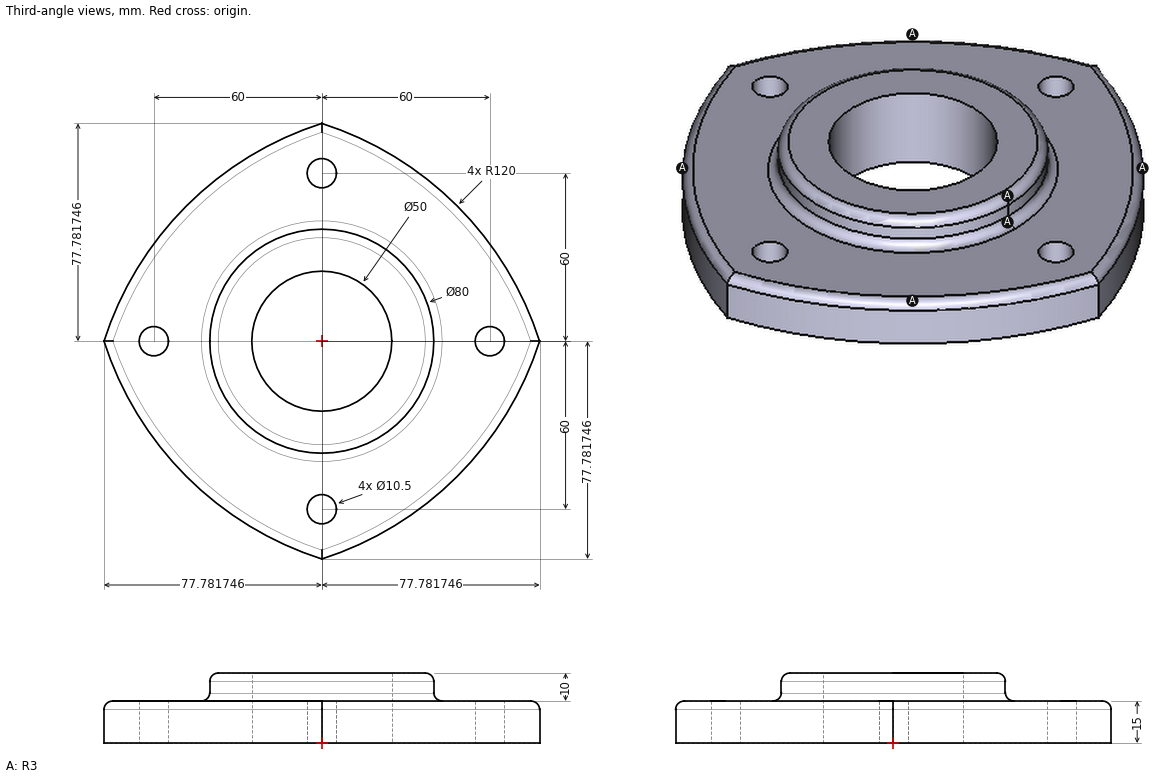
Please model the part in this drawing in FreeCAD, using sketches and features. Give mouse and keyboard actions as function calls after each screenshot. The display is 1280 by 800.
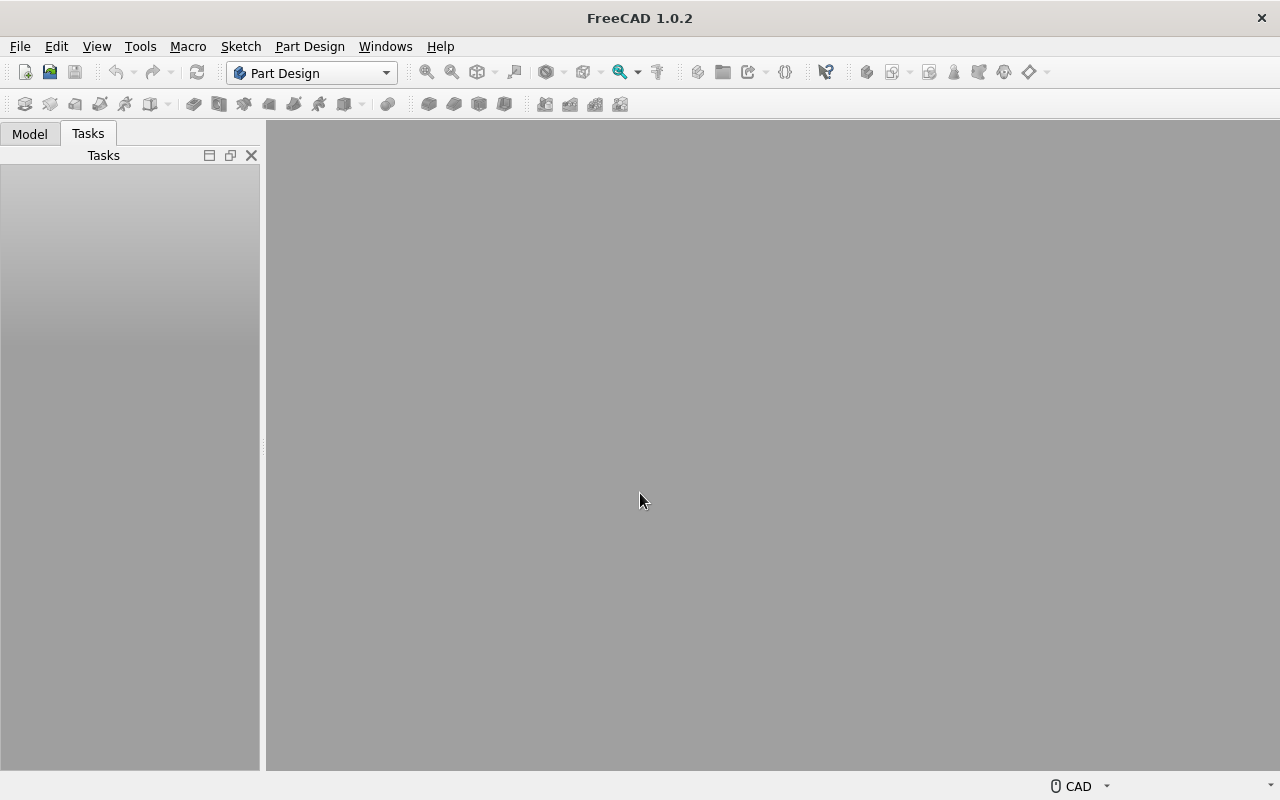
click(25, 72)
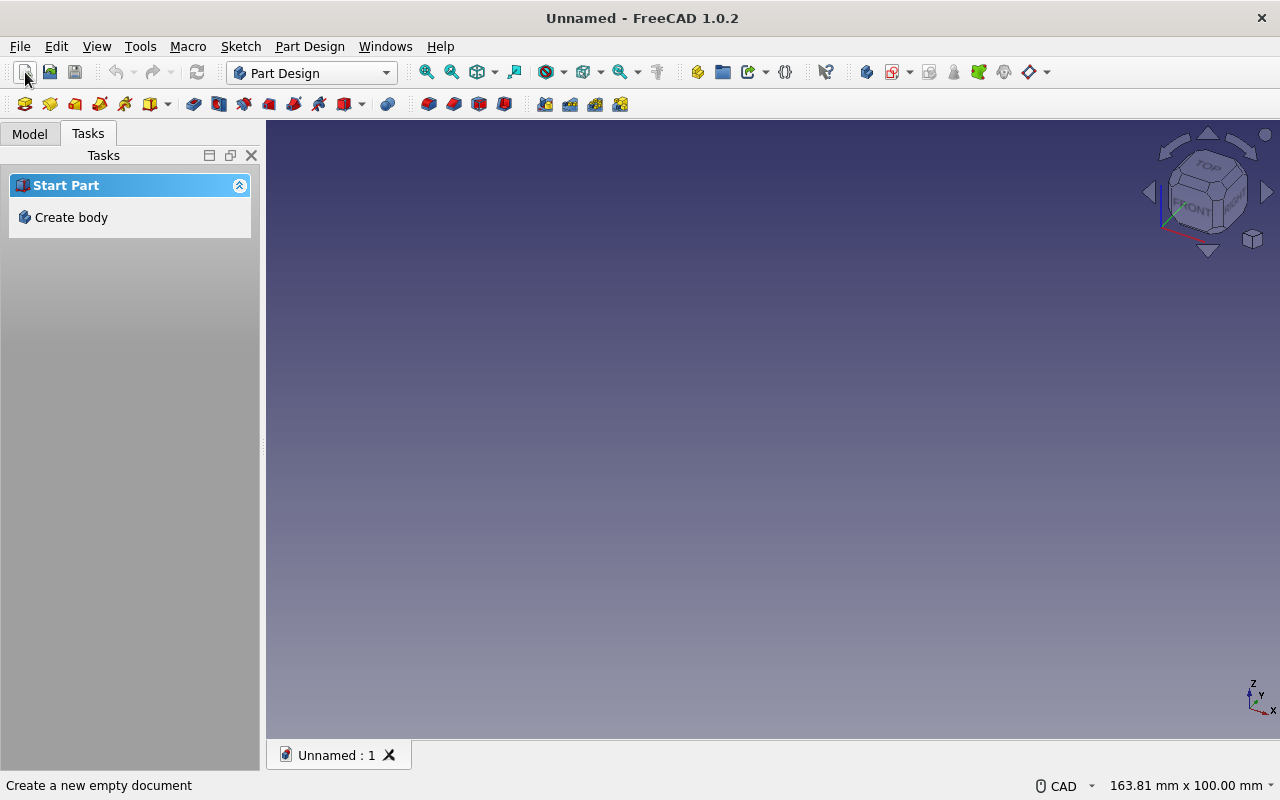
click(892, 72)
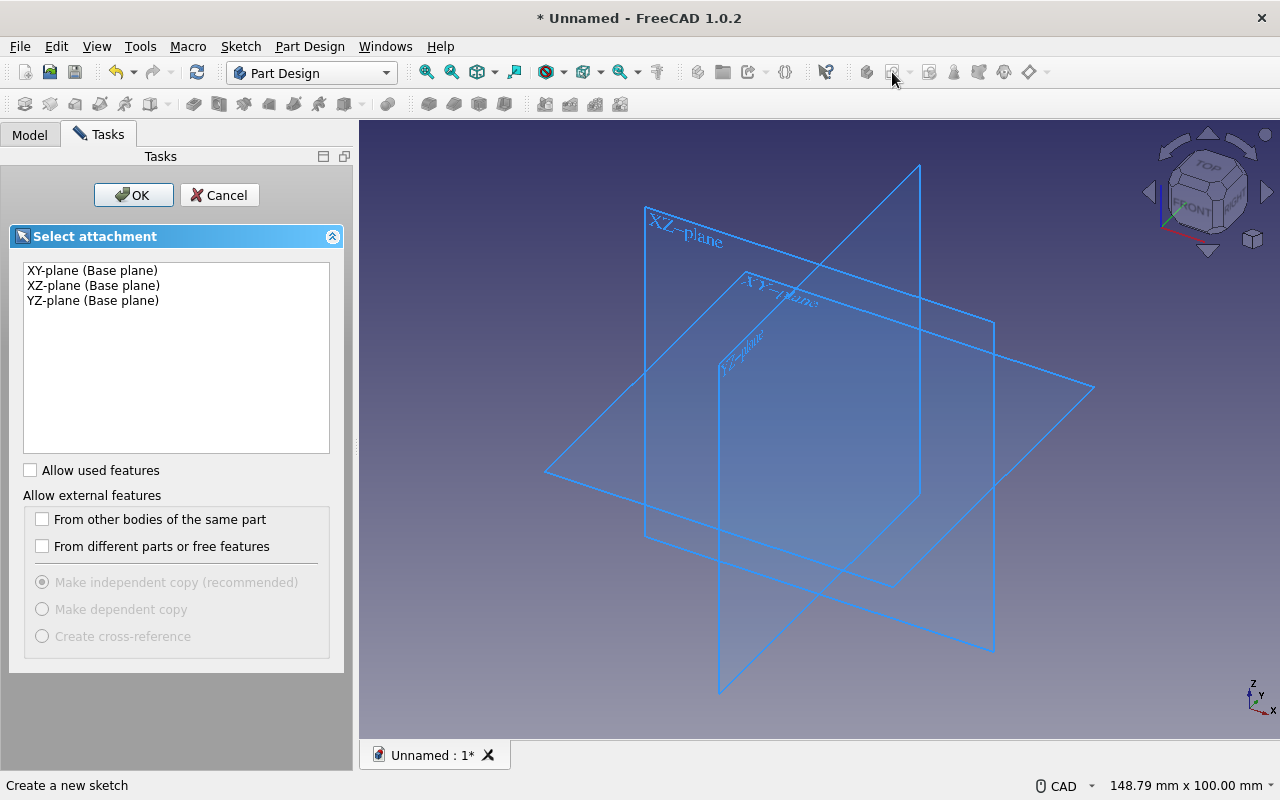
click(84, 270)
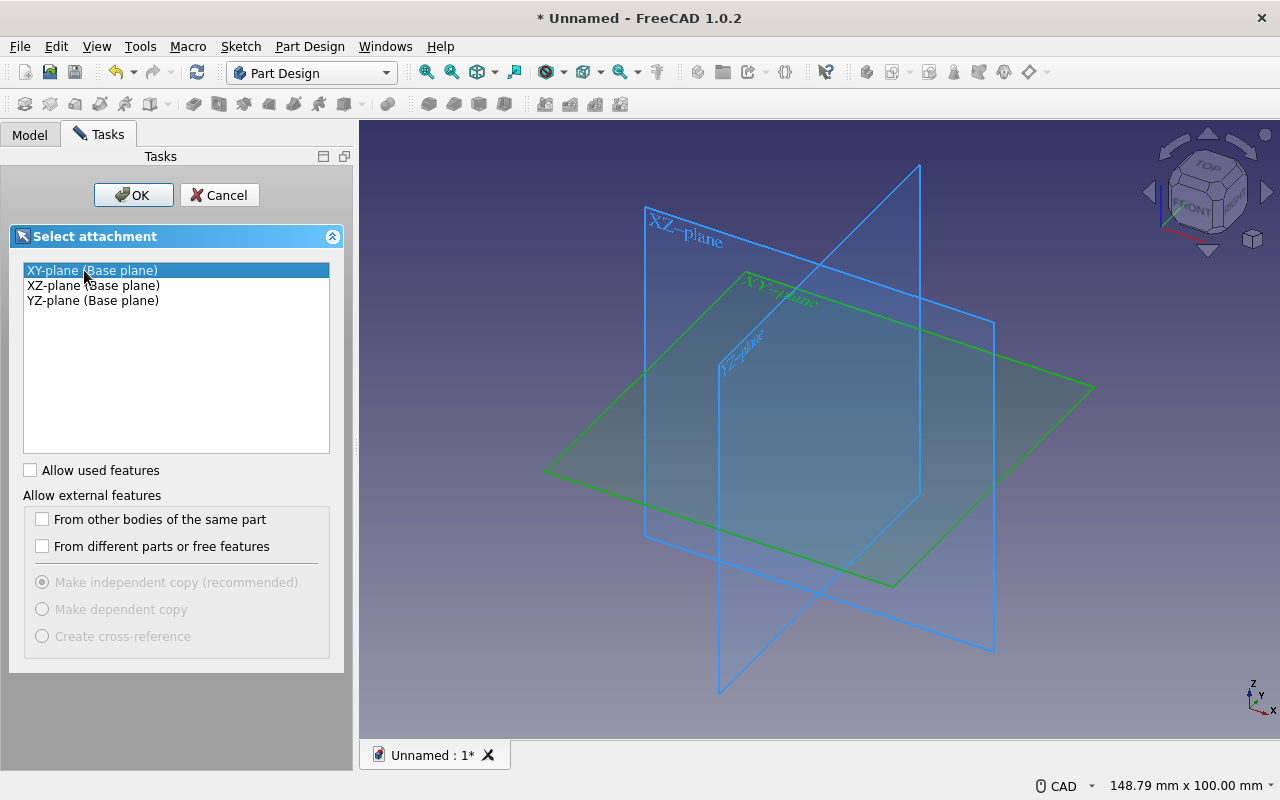
click(134, 195)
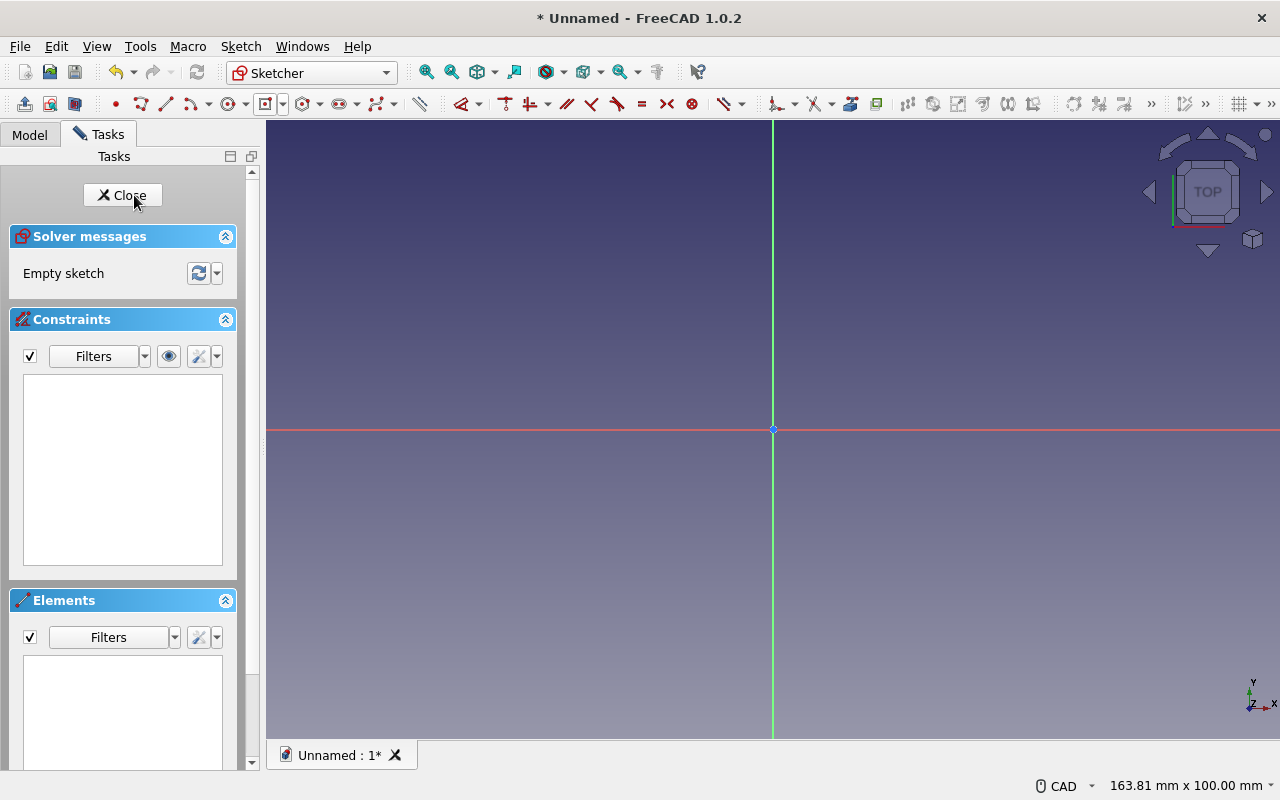
scroll(649, 430, down, 4)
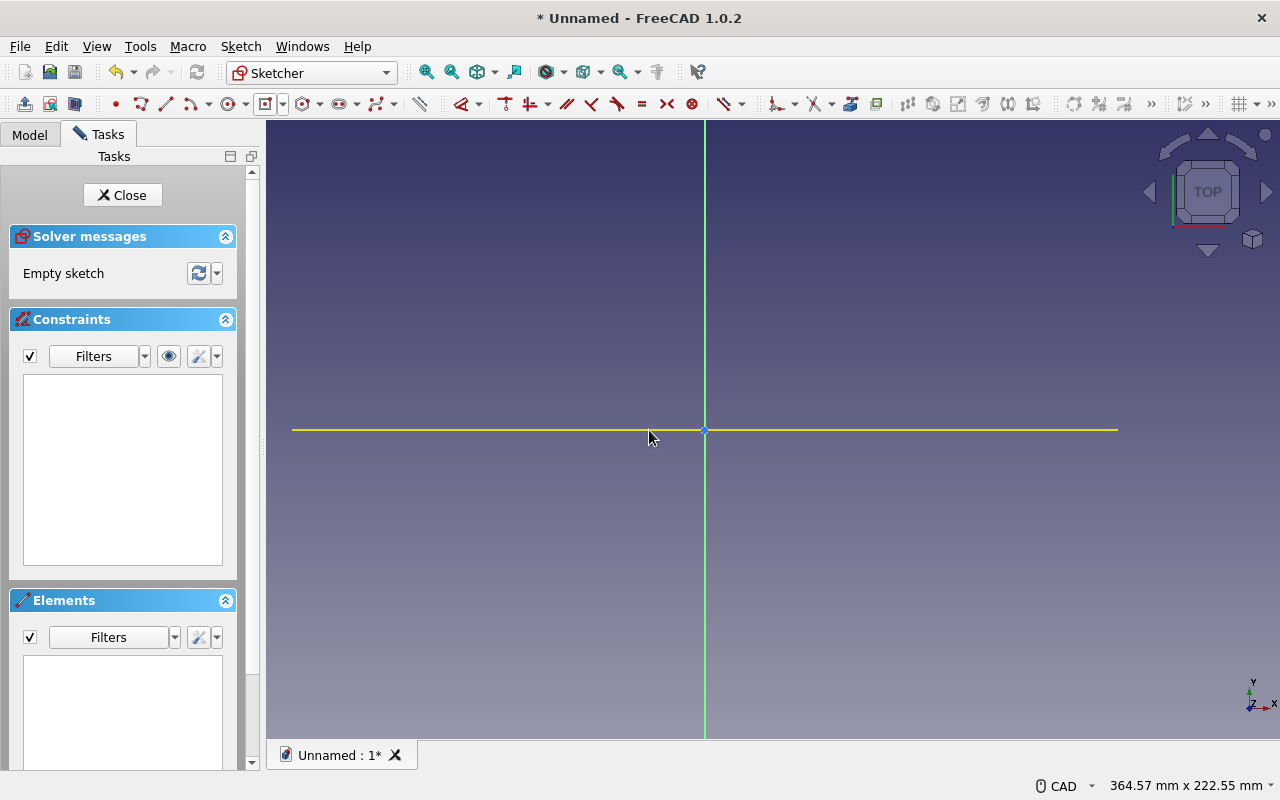
key(g)
key(3)
key(a)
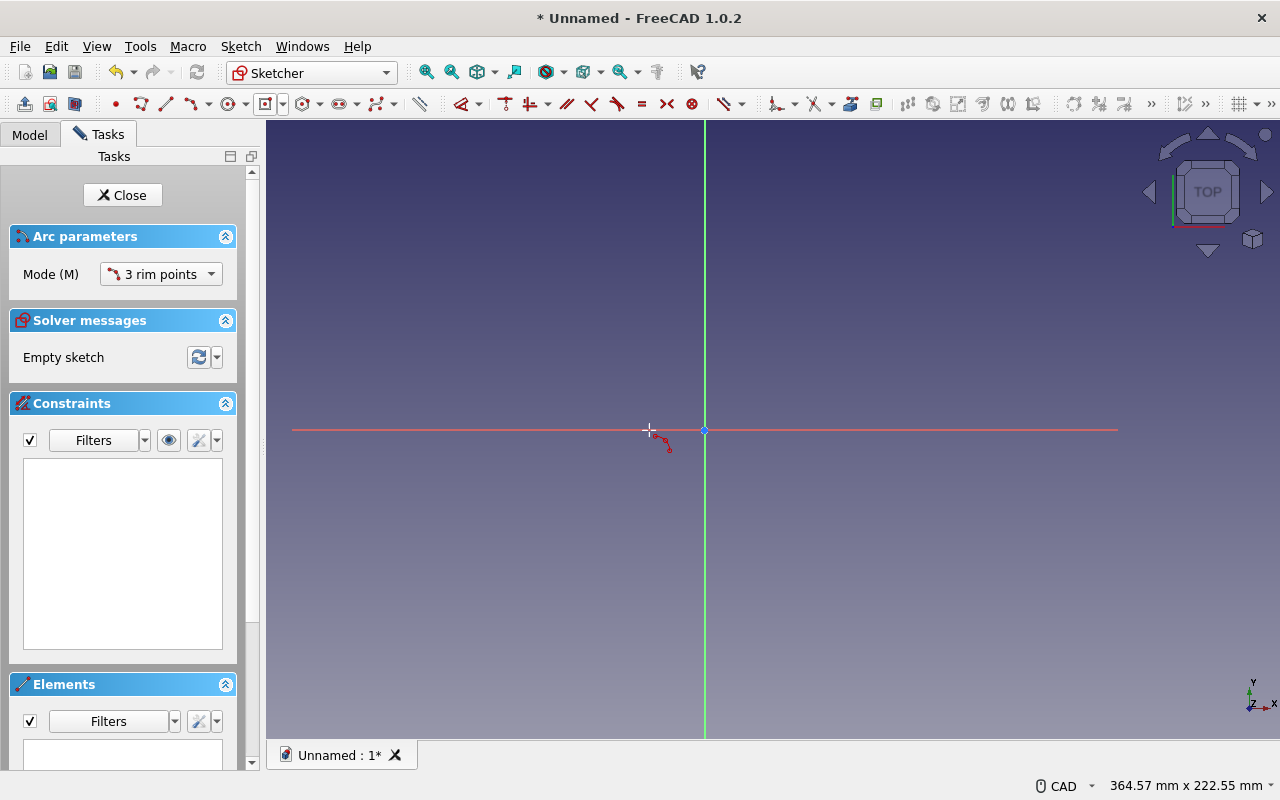
click(921, 430)
click(705, 214)
click(839, 296)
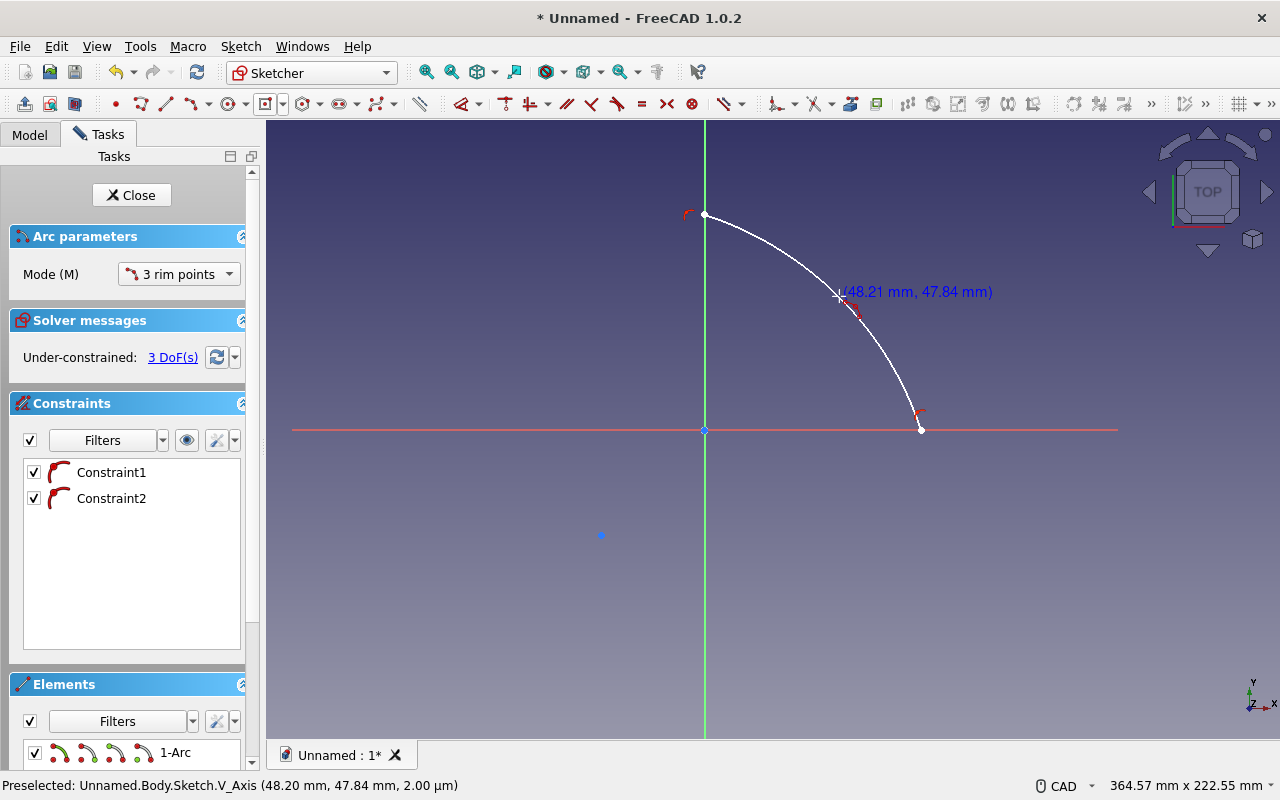
click(705, 215)
click(489, 430)
click(571, 296)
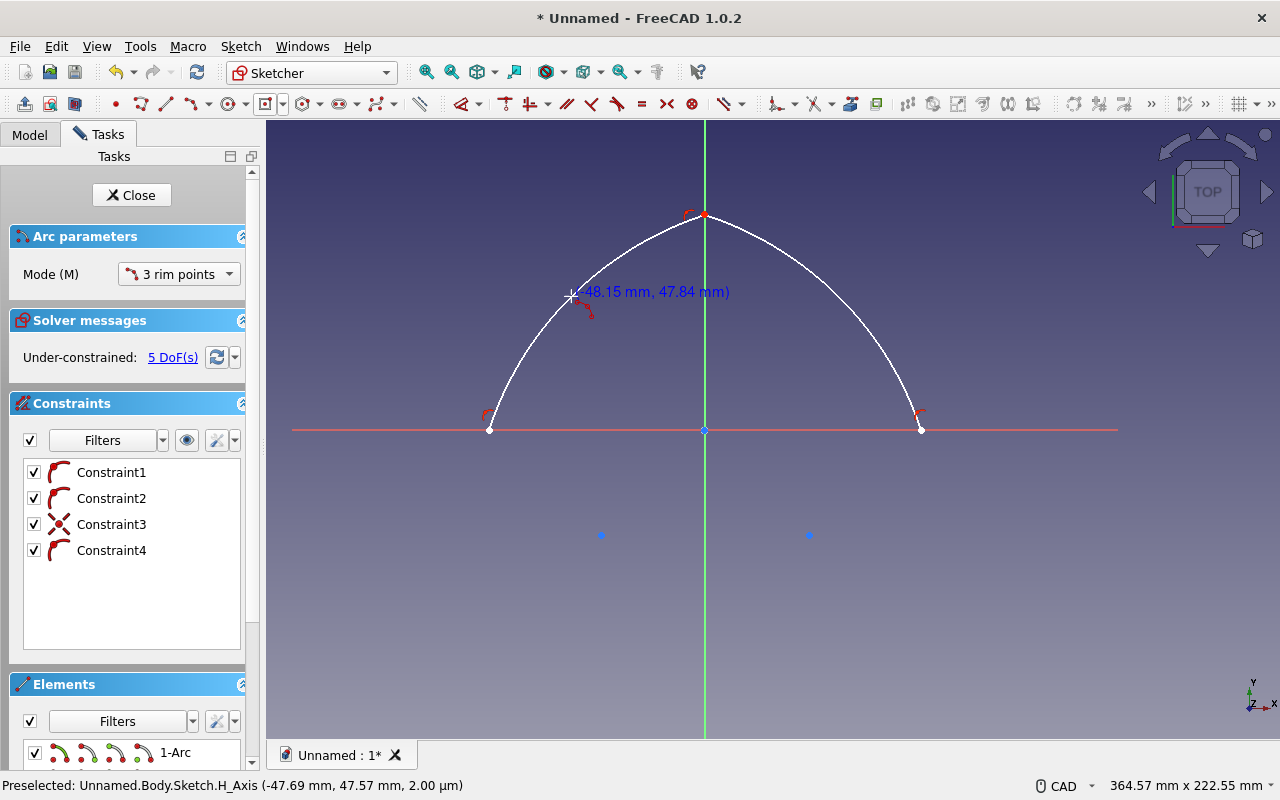
click(489, 430)
click(705, 646)
click(571, 564)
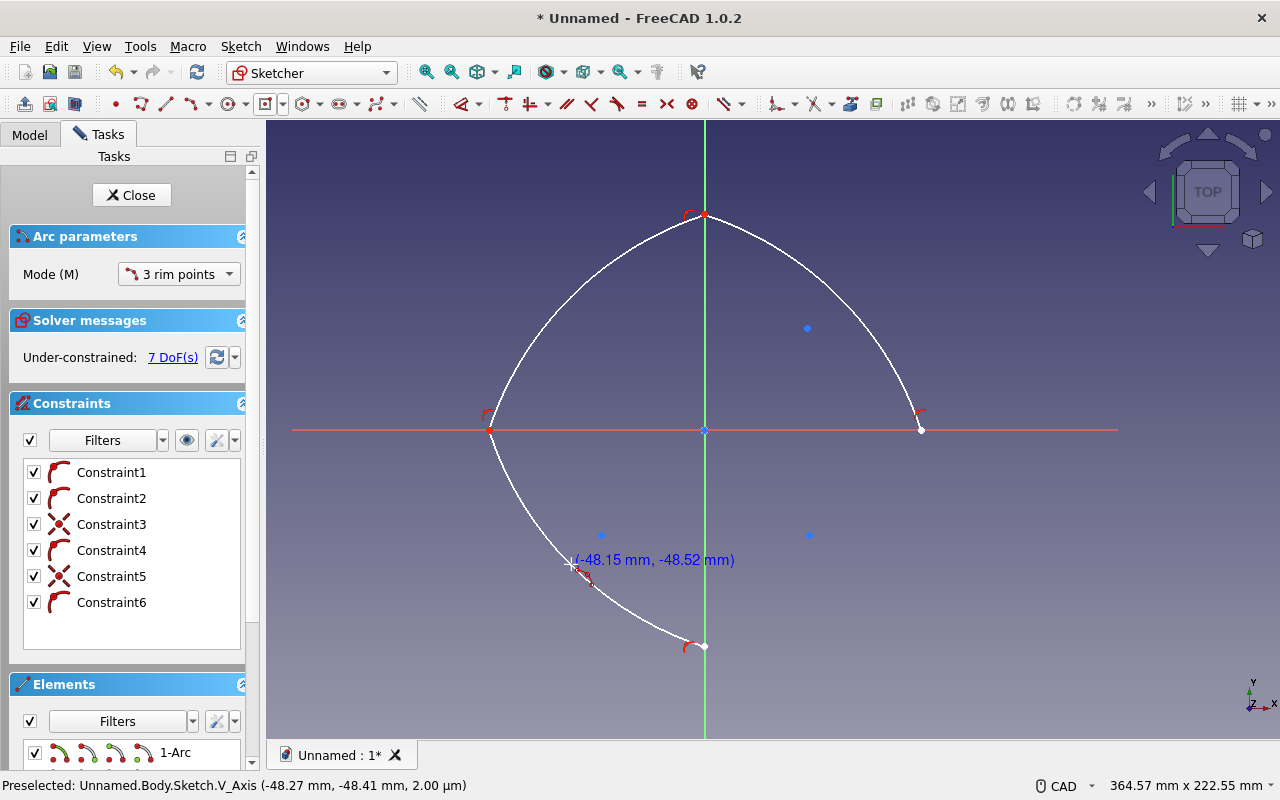
click(705, 647)
click(921, 430)
click(839, 564)